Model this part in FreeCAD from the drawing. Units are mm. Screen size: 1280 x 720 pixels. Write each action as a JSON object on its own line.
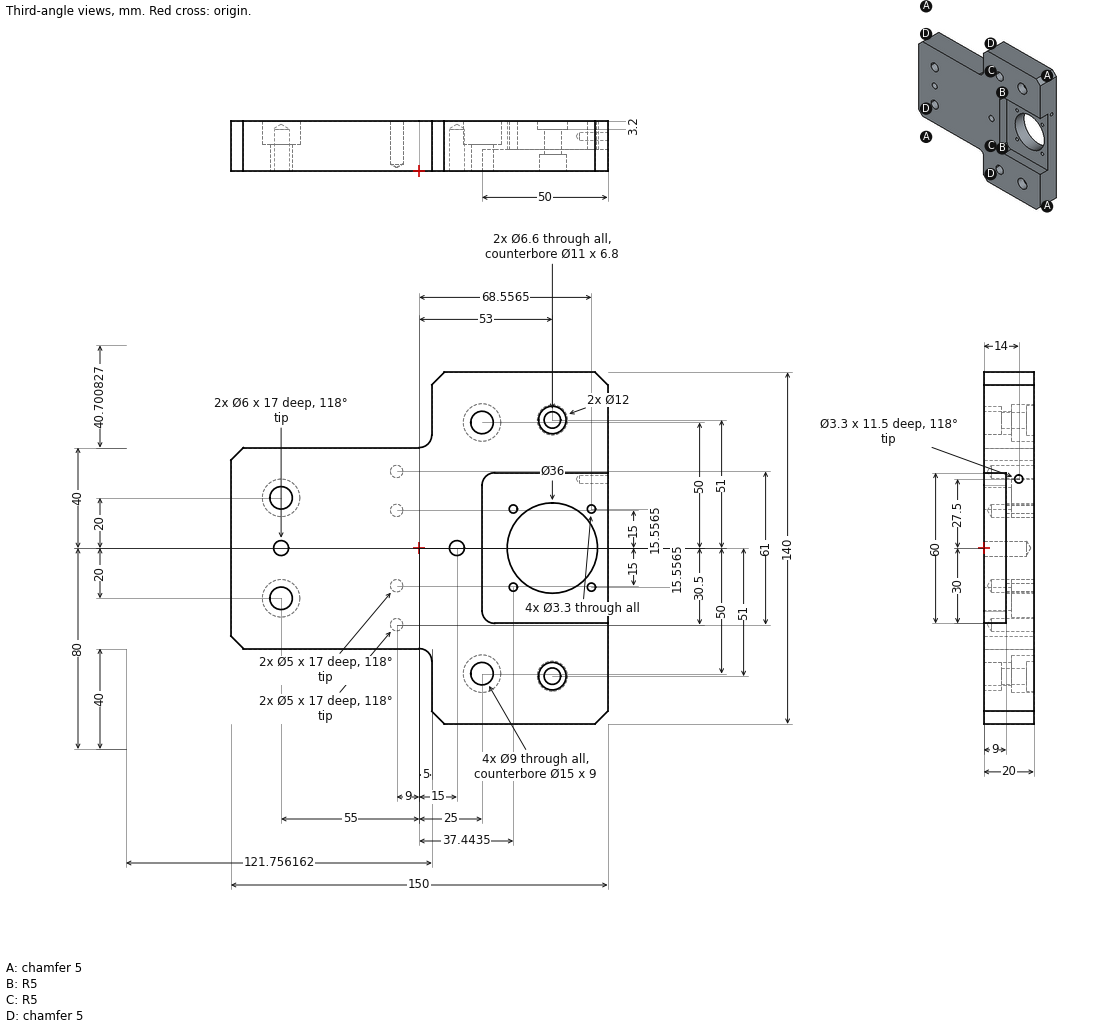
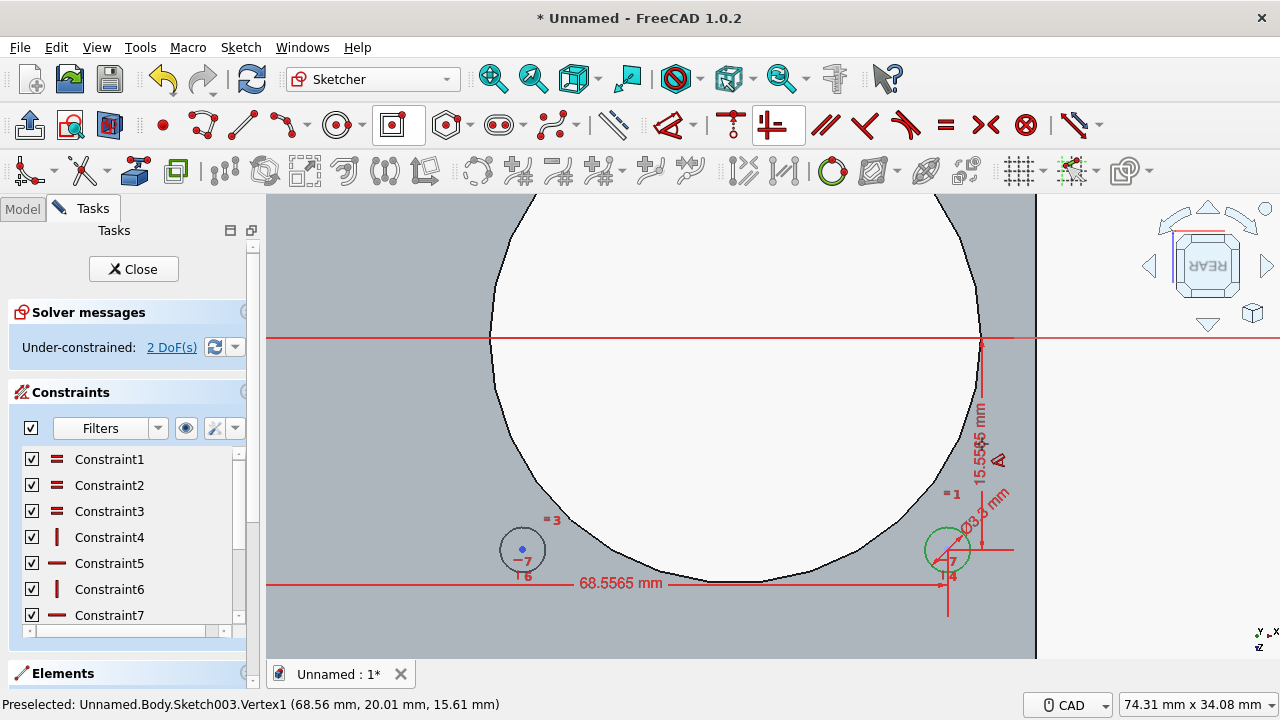
{"action": "scroll", "coordinate": [964, 535], "scroll_direction": "down", "scroll_amount": 3}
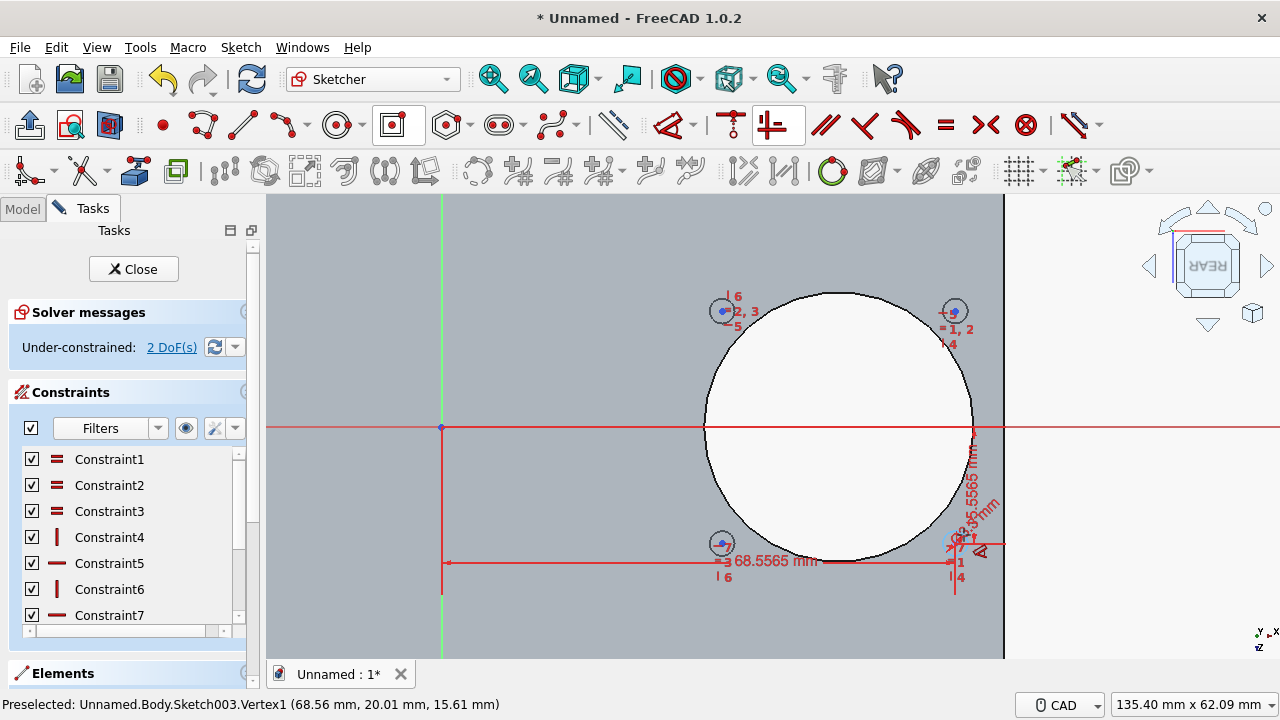
{"action": "left_click", "coordinate": [955, 311]}
{"action": "left_click", "coordinate": [408, 369]}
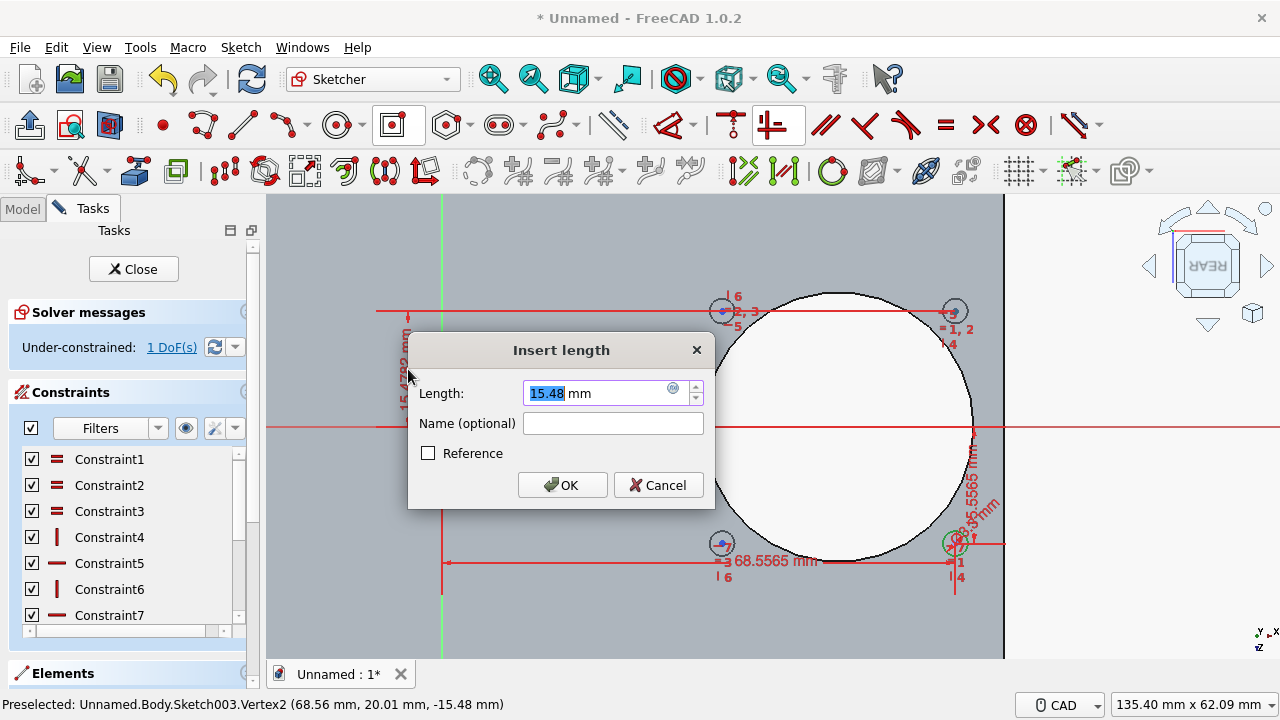
{"action": "type", "text": "15.5565"}
{"action": "key", "text": "Return"}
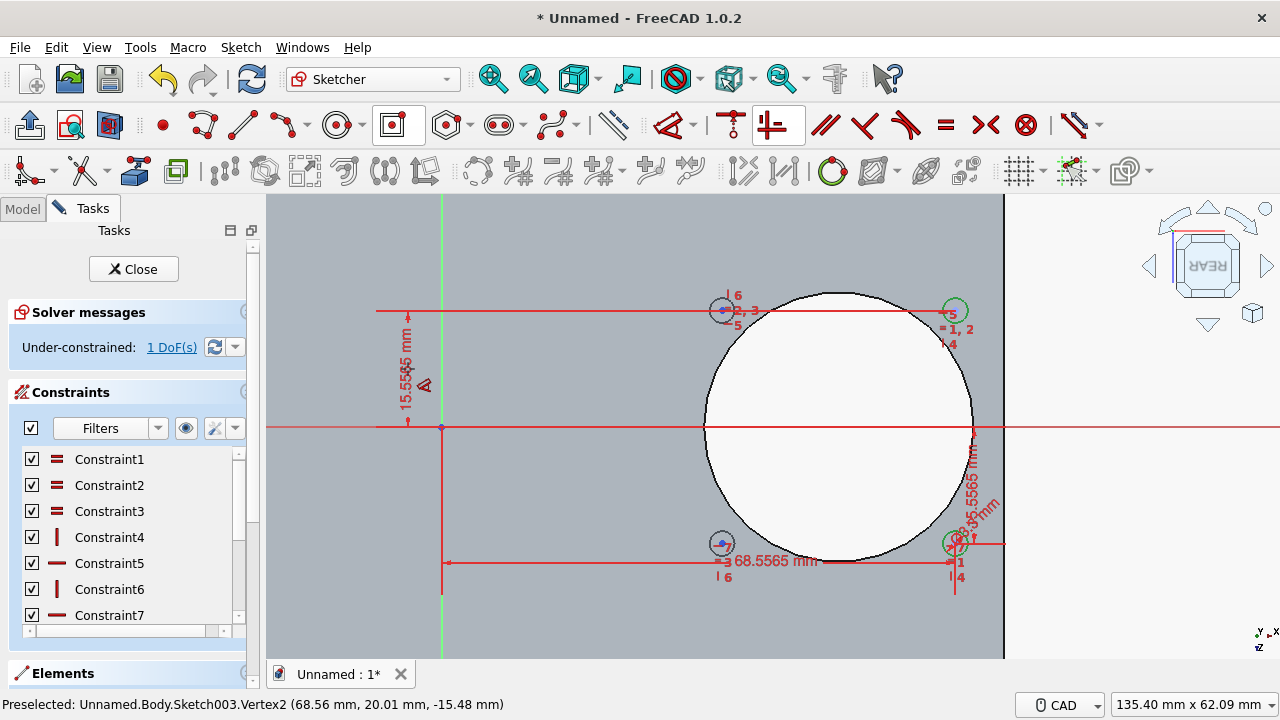
{"action": "left_click", "coordinate": [722, 311]}
{"action": "left_click", "coordinate": [582, 277]}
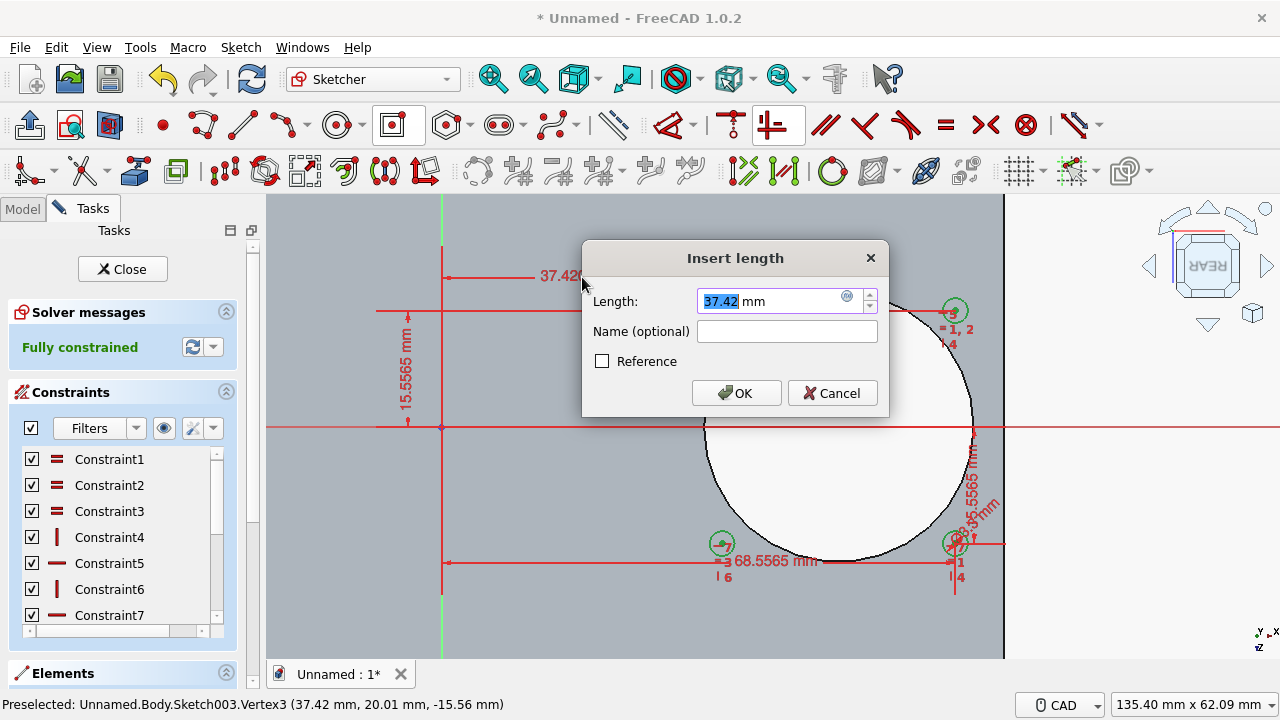
{"action": "type", "text": "37.4435"}
{"action": "key", "text": "Return"}
{"action": "key", "text": "Escape"}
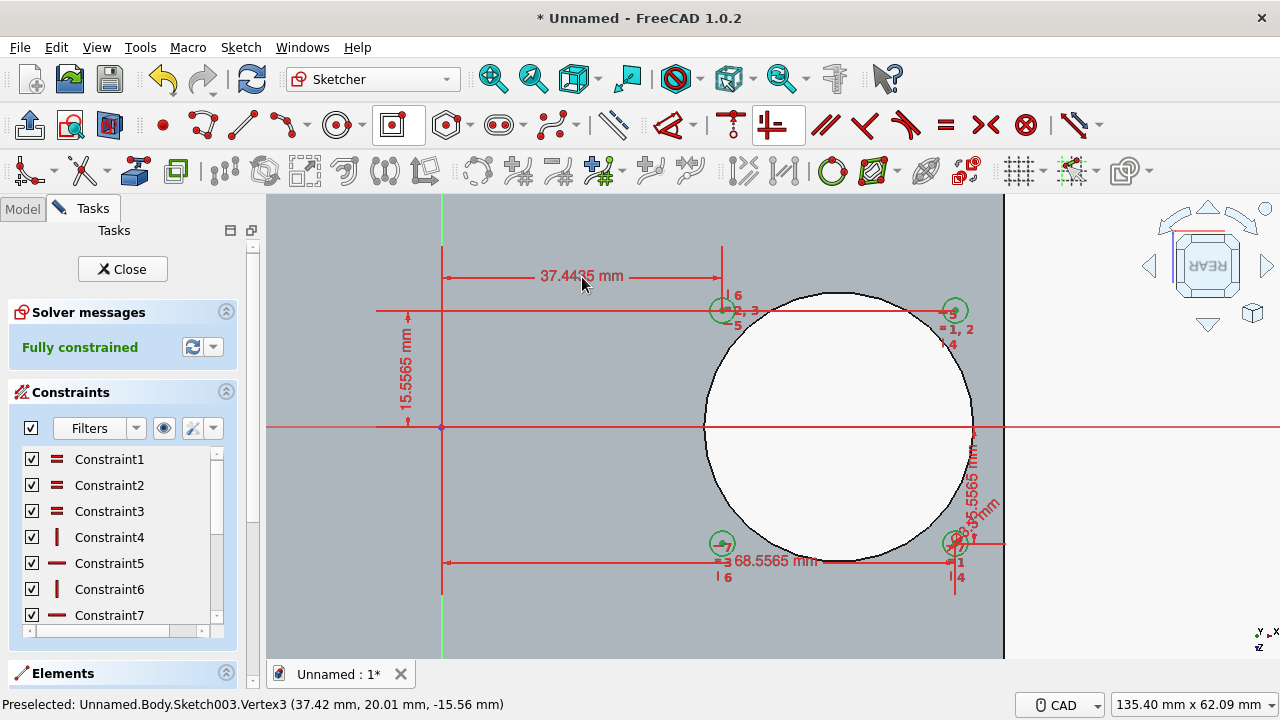
{"action": "left_click", "coordinate": [123, 269]}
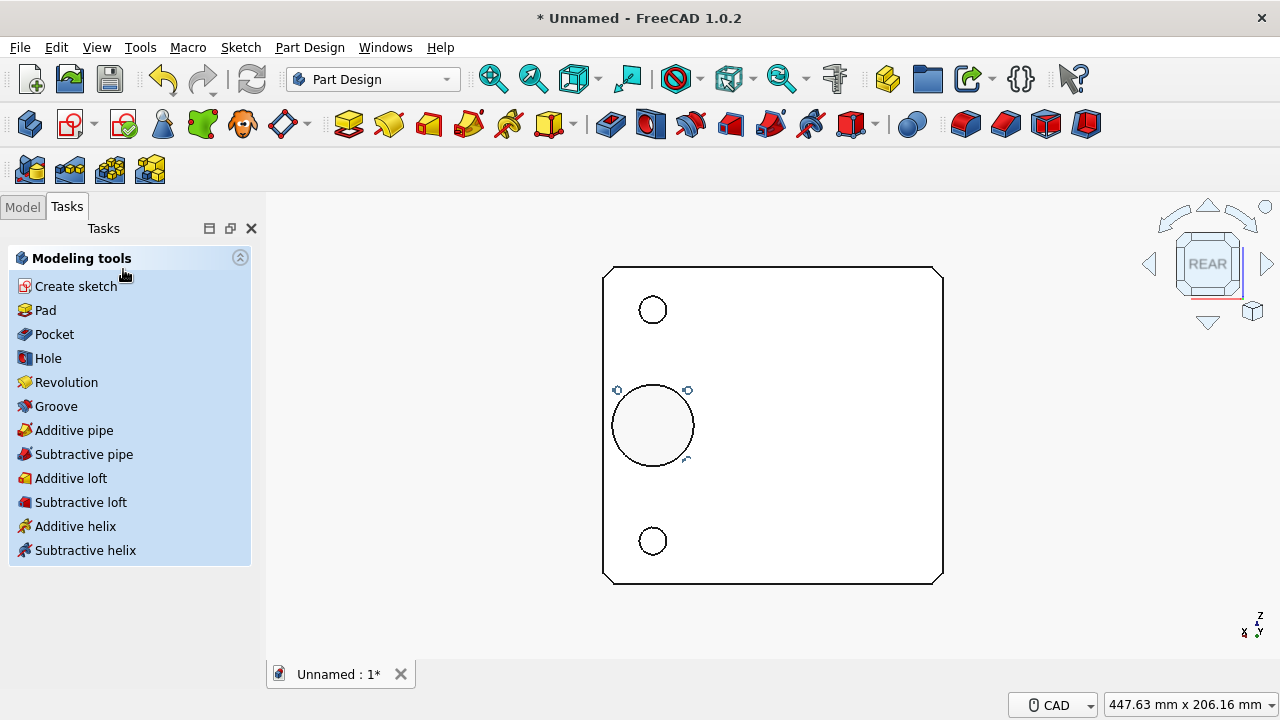
{"action": "left_click", "coordinate": [652, 124]}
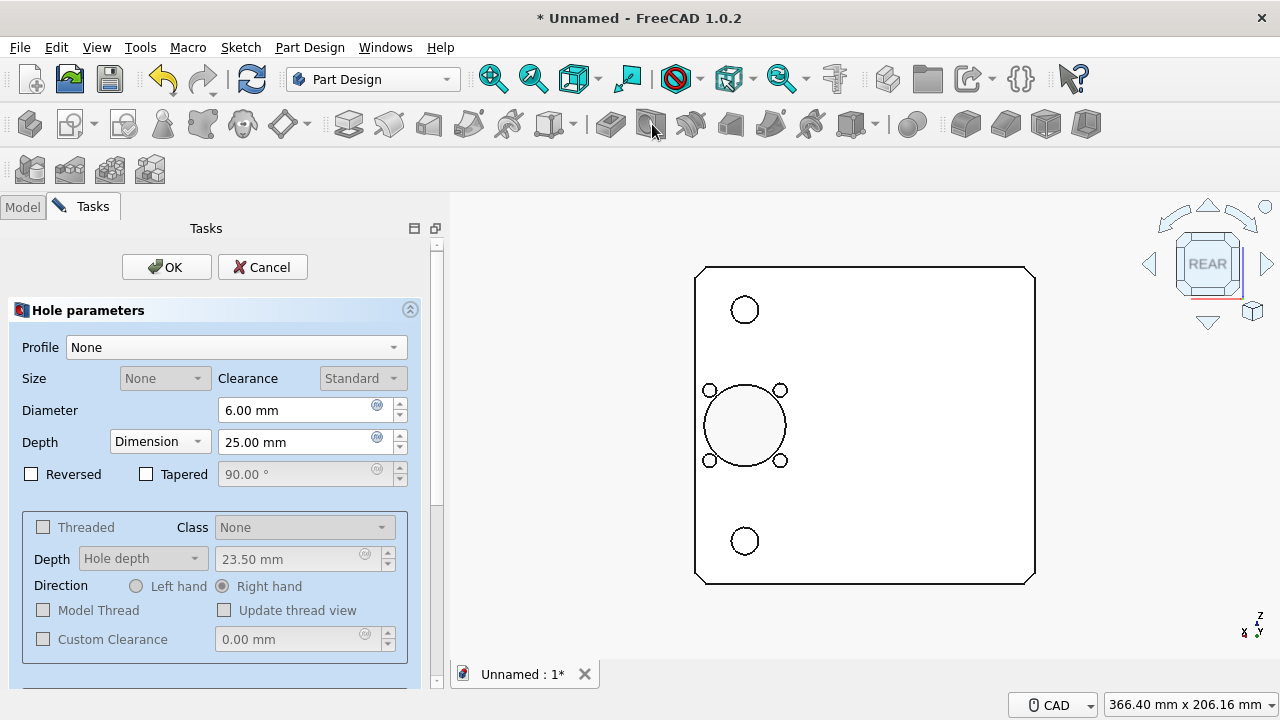
{"action": "triple_click", "coordinate": [305, 410]}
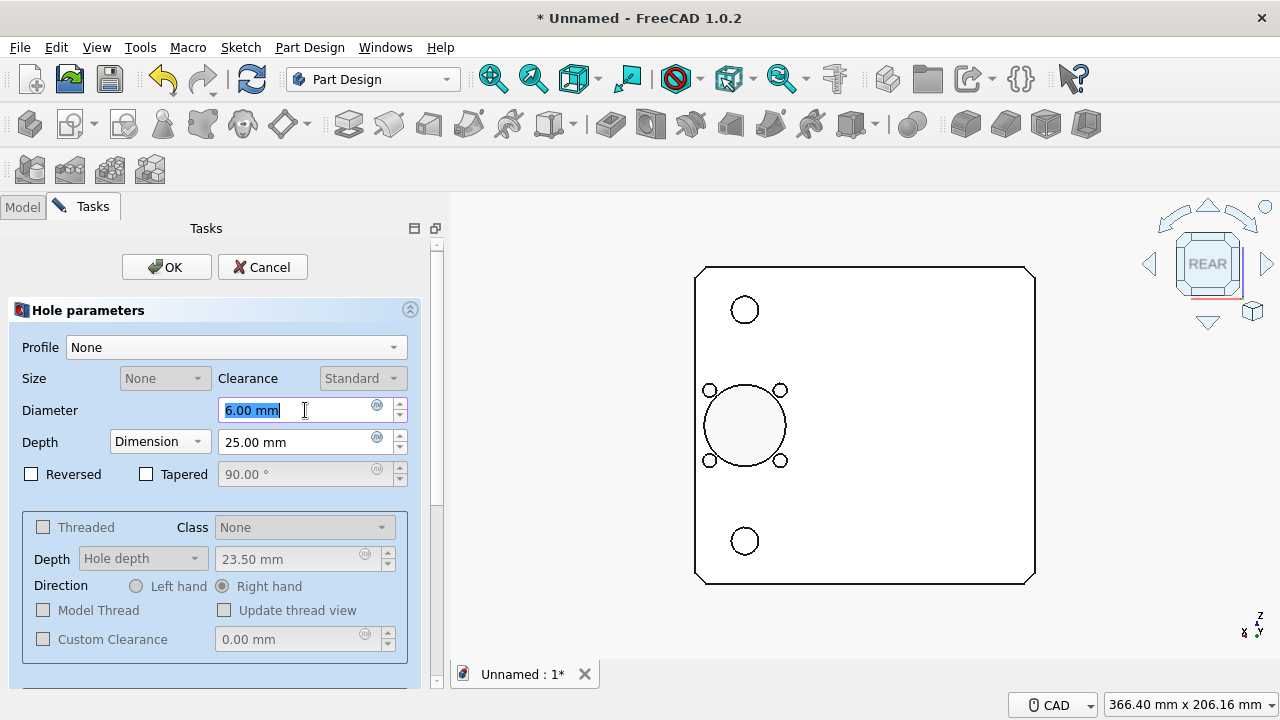
{"action": "type", "text": "3.3"}
{"action": "key", "text": "Tab"}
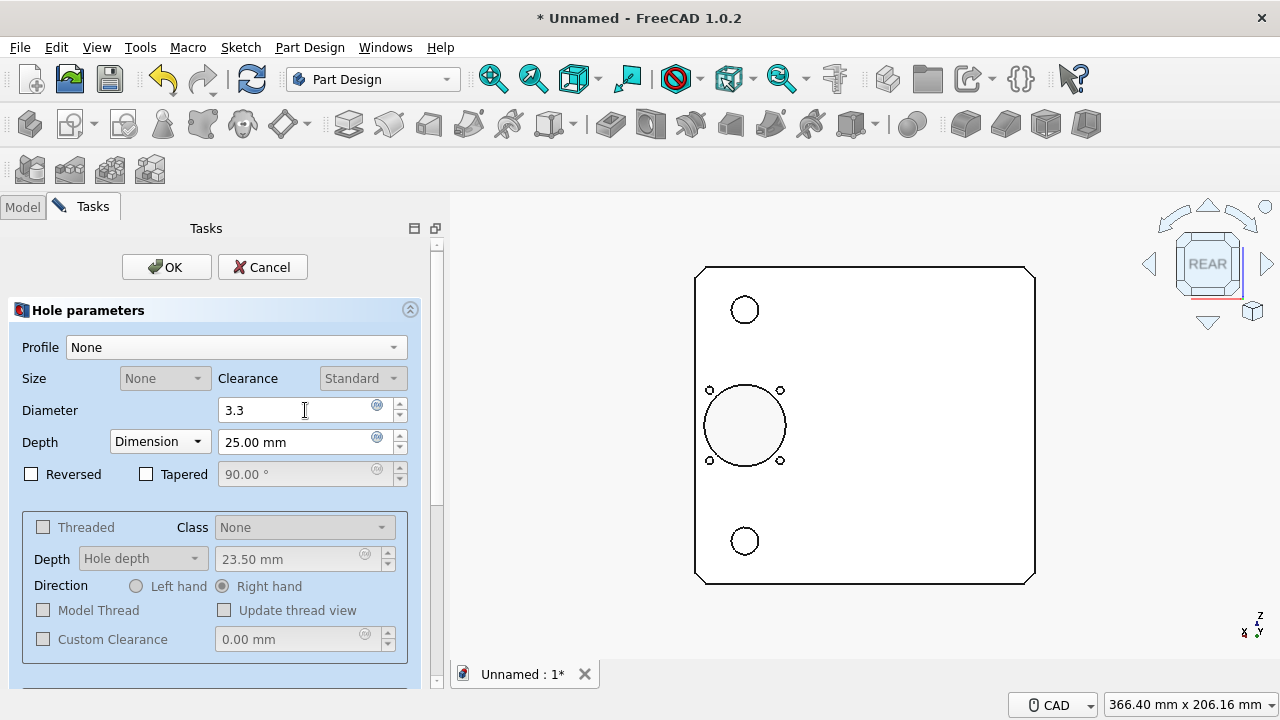
{"action": "left_click", "coordinate": [161, 442]}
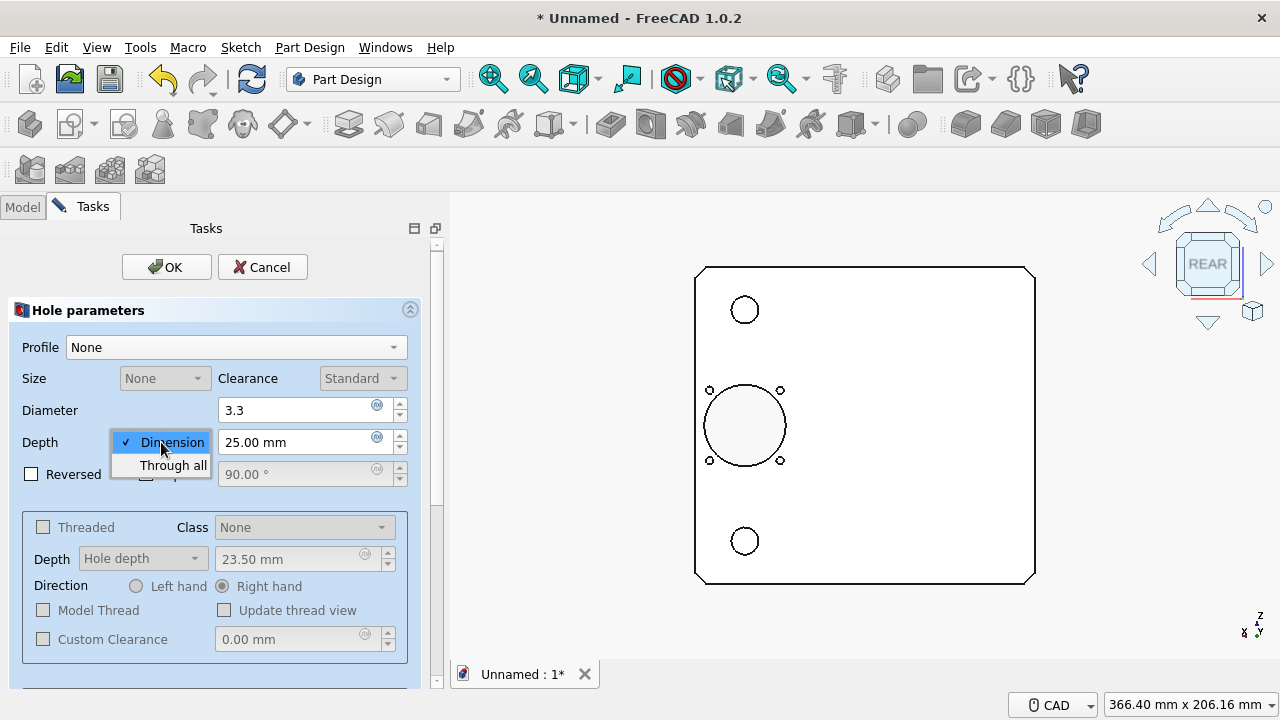
{"action": "left_click", "coordinate": [160, 466]}